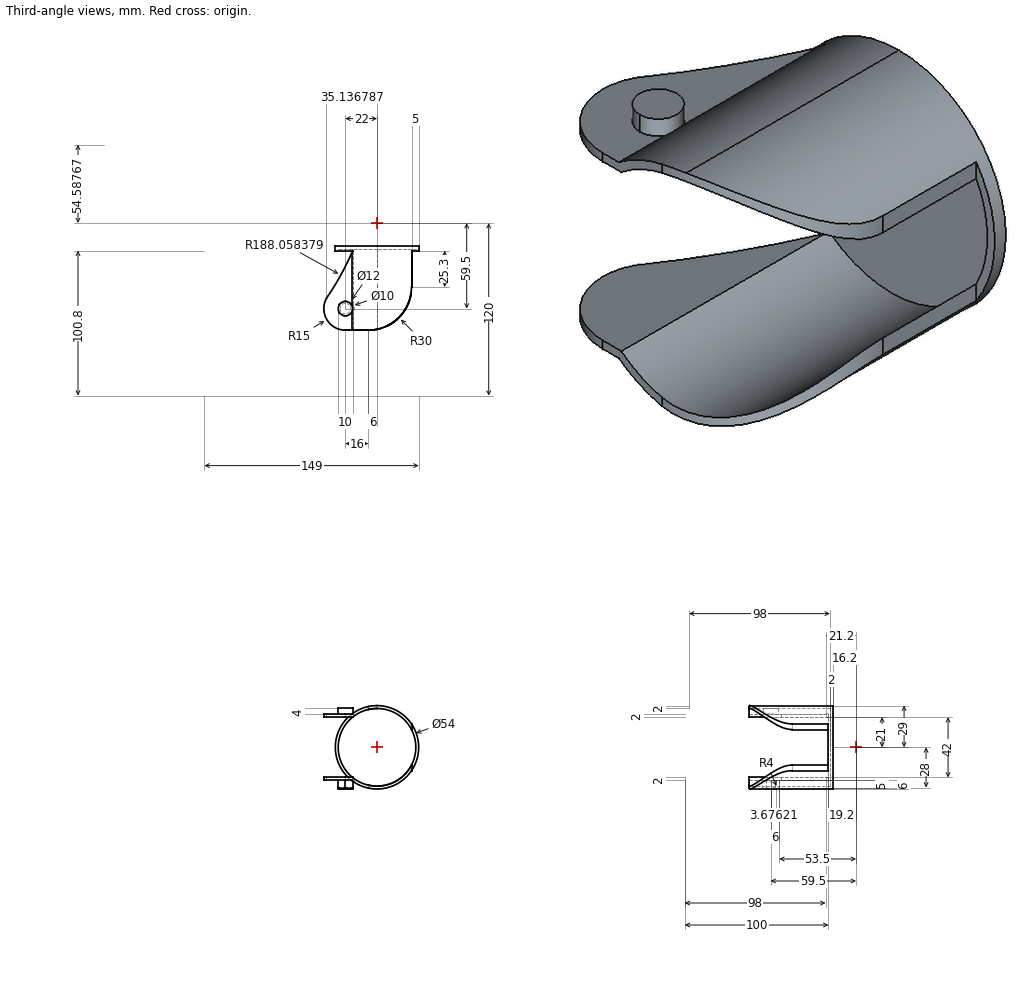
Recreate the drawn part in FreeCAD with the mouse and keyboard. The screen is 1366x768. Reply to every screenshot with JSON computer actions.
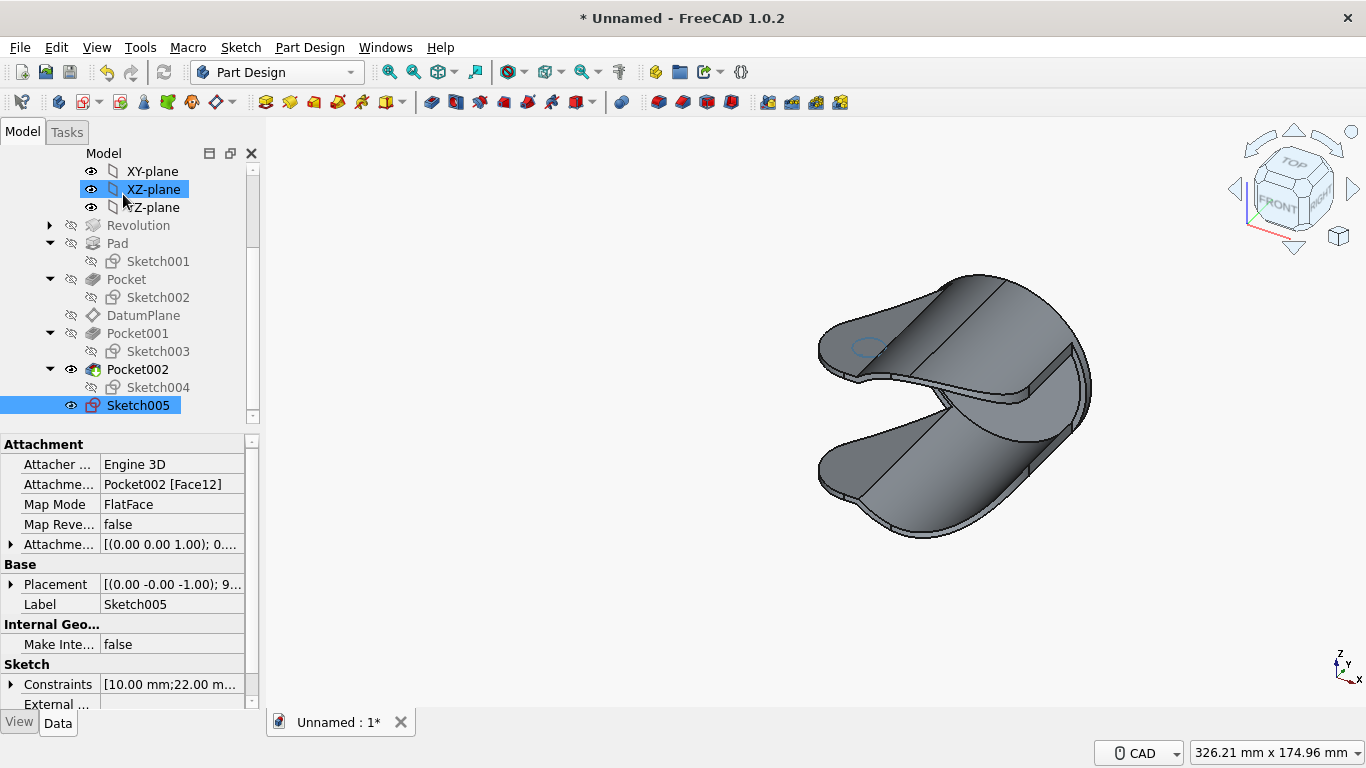
{"action": "left_click", "coordinate": [266, 102]}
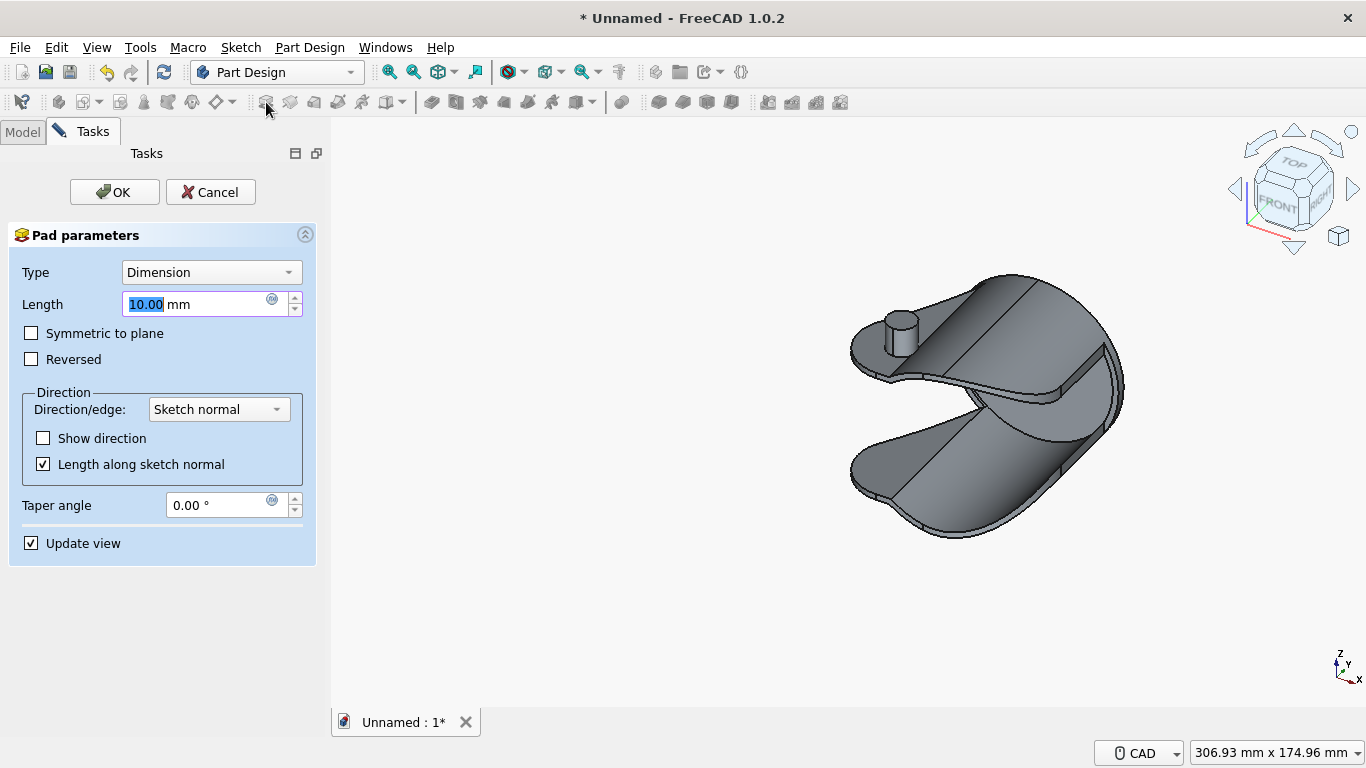
{"action": "type", "text": "4"}
{"action": "key", "text": "Tab"}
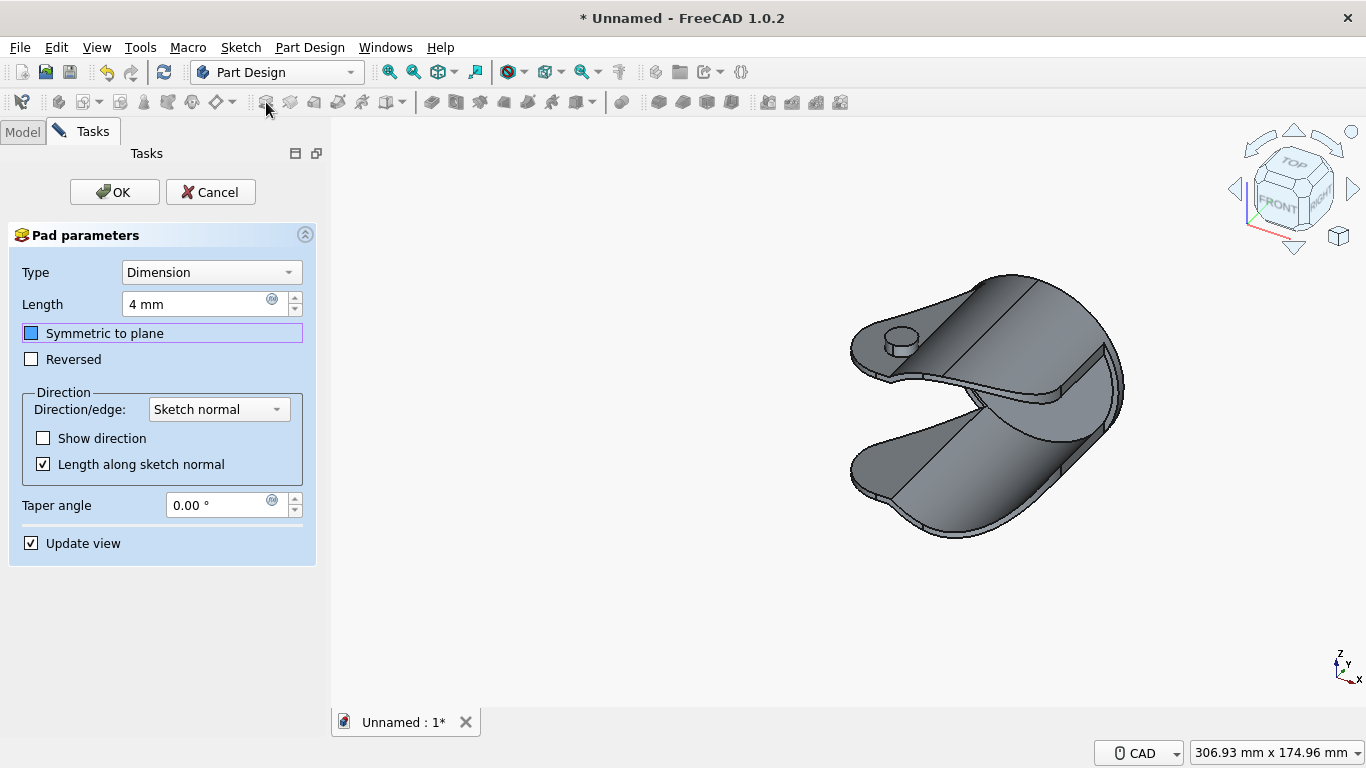
{"action": "left_click", "coordinate": [115, 192]}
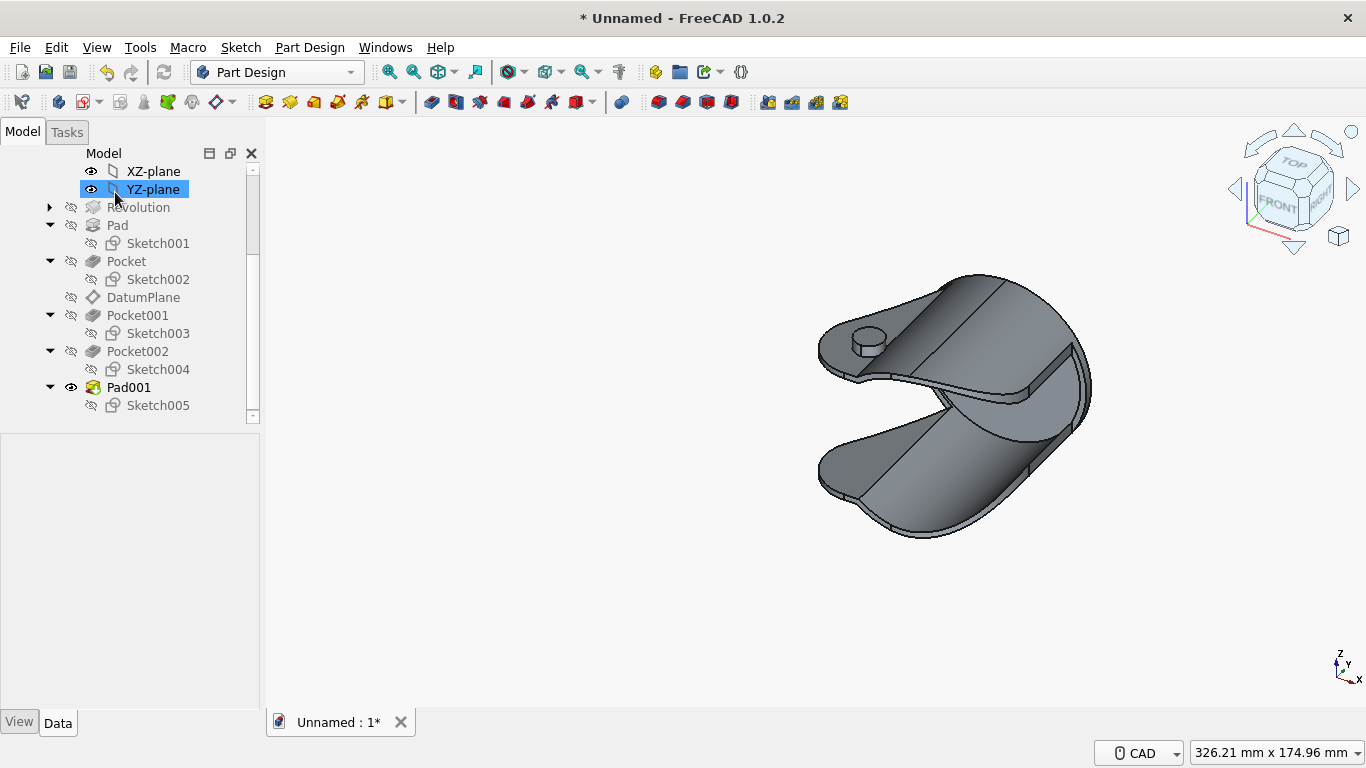
{"action": "scroll", "coordinate": [160, 293], "scroll_direction": "down", "scroll_amount": 3}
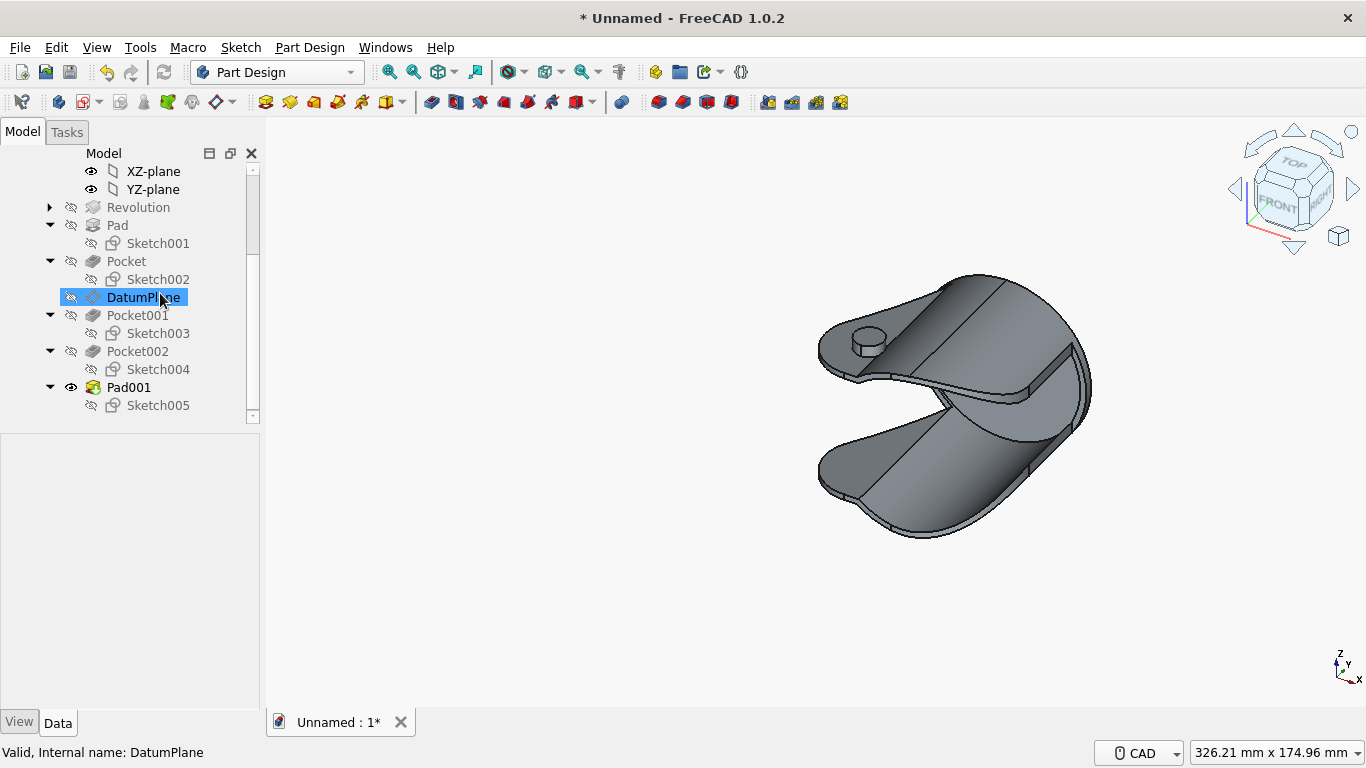
{"action": "scroll", "coordinate": [160, 293], "scroll_direction": "up", "scroll_amount": 15}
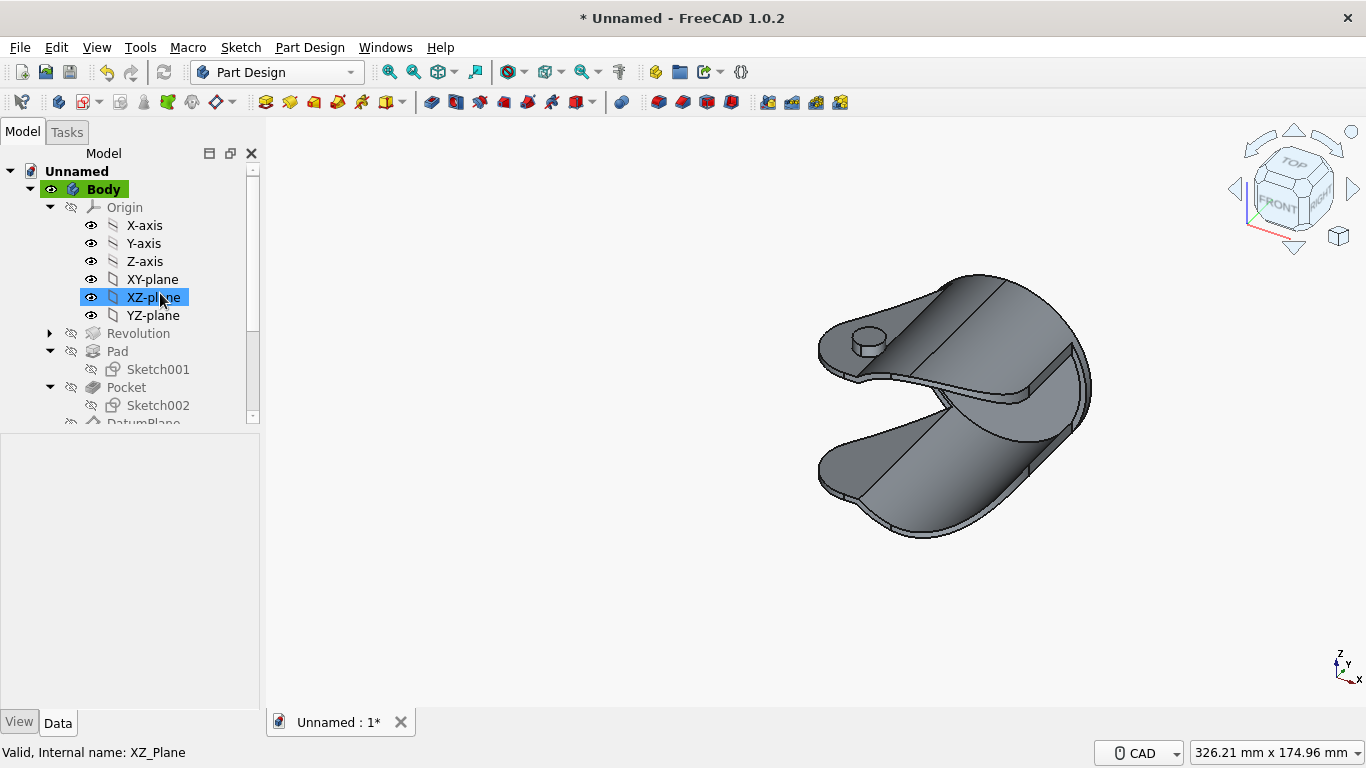
{"action": "left_click", "coordinate": [136, 315]}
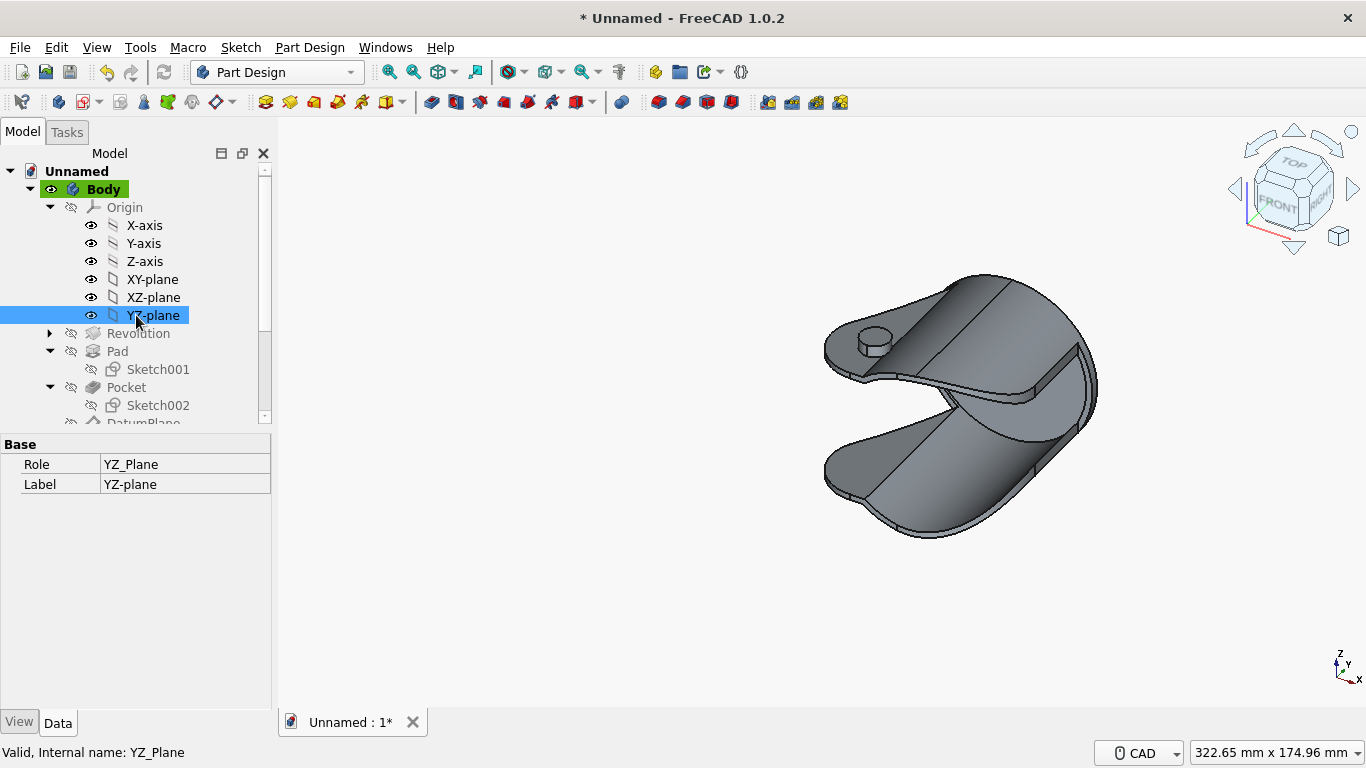
{"action": "left_click", "coordinate": [216, 102]}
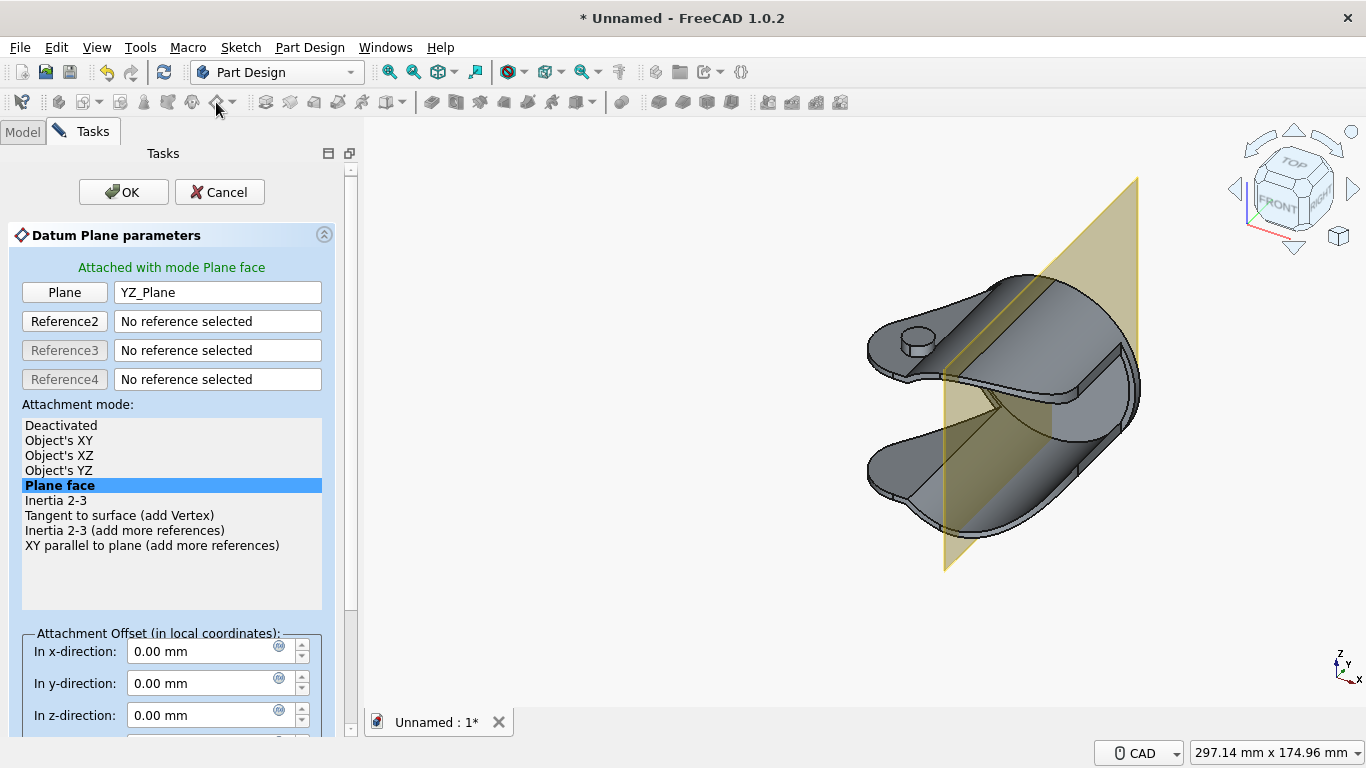
{"action": "triple_click", "coordinate": [210, 715]}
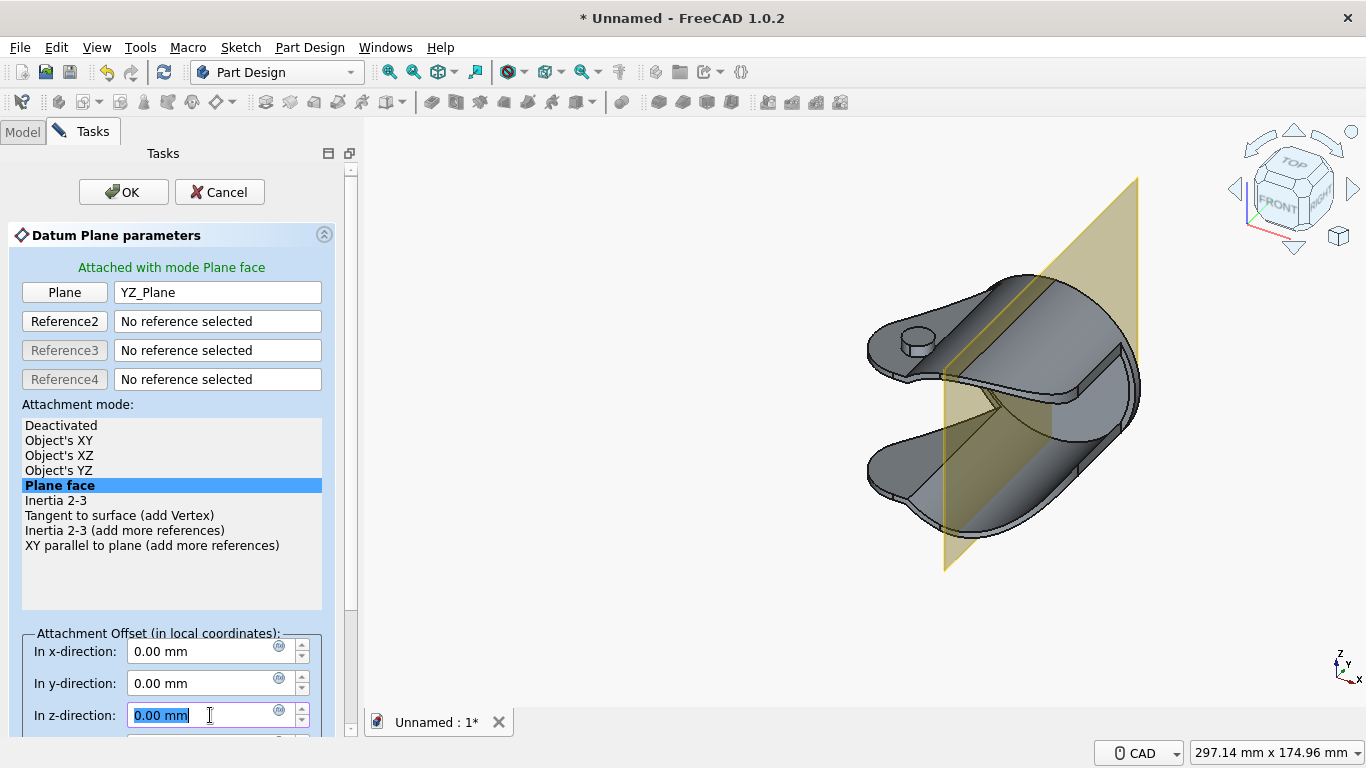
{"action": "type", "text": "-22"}
{"action": "key", "text": "Tab"}